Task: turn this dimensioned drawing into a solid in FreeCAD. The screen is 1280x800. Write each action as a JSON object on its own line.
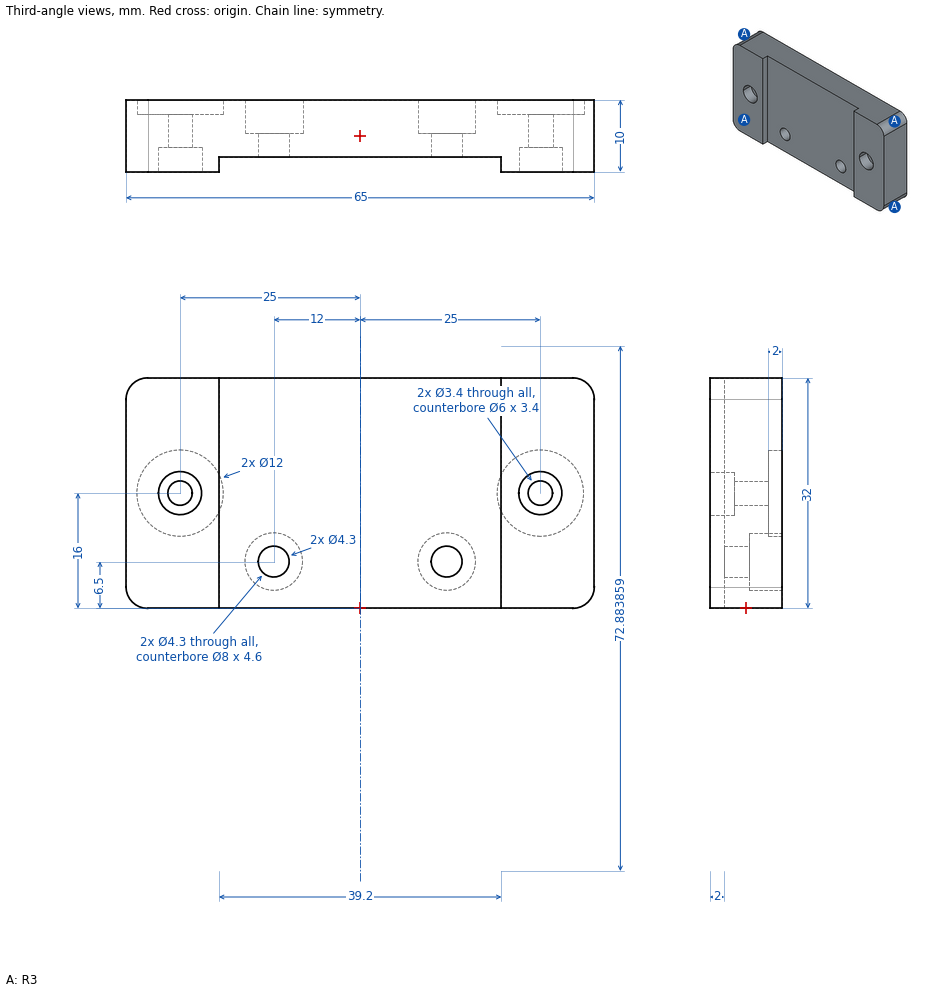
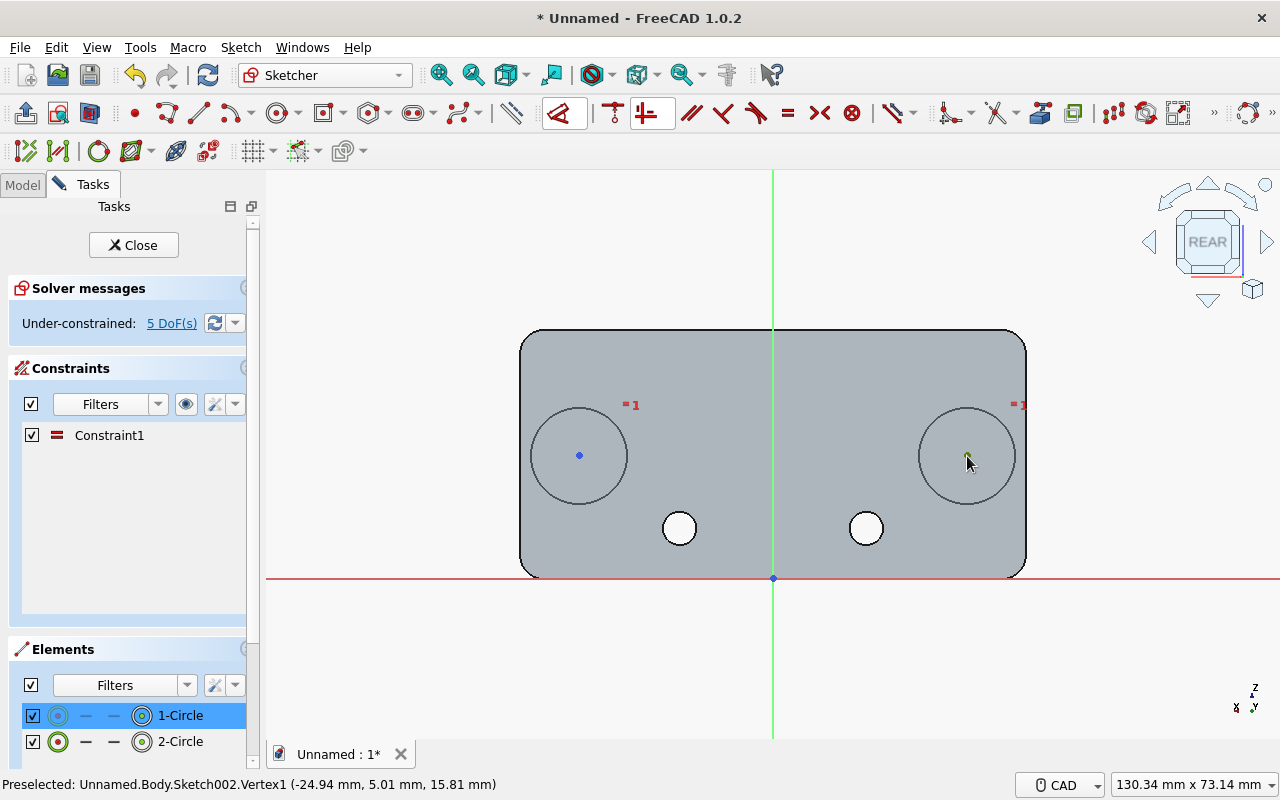
{"action": "left_click", "coordinate": [579, 456]}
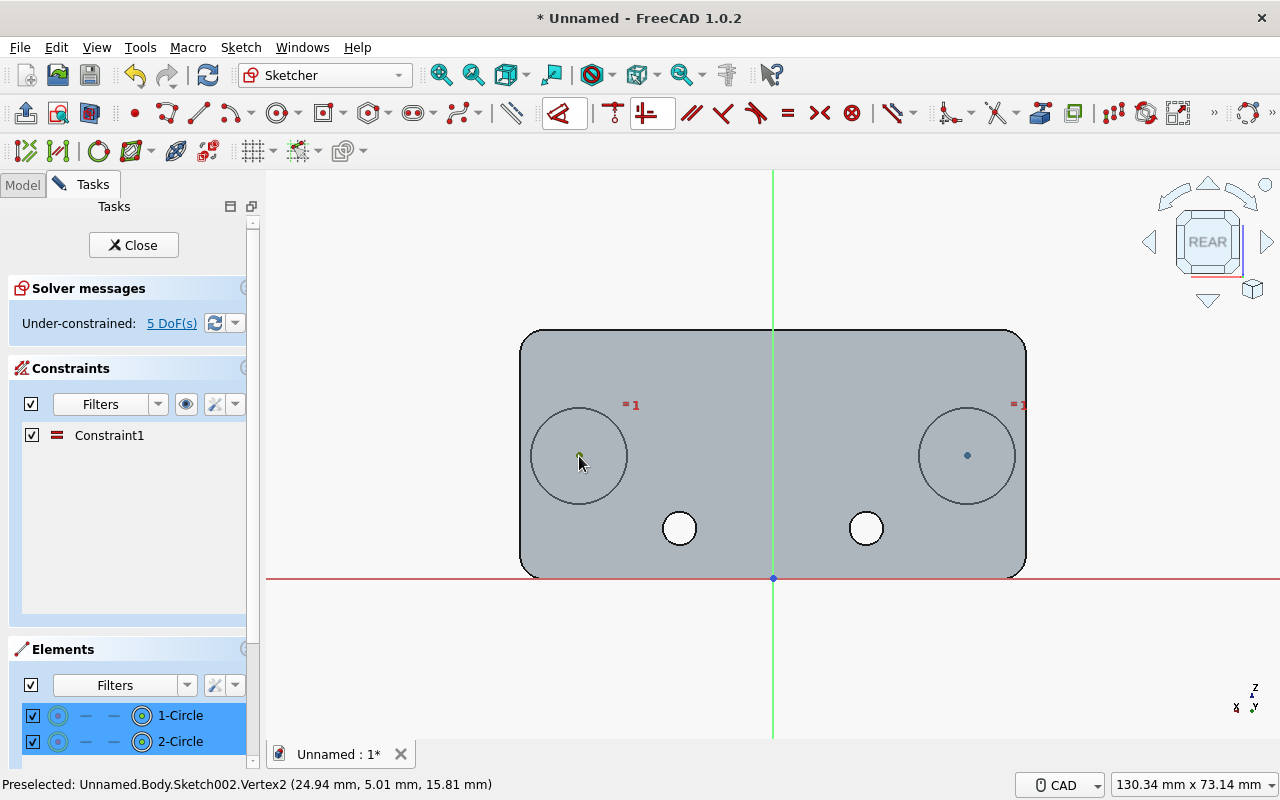
{"action": "left_click", "coordinate": [773, 674]}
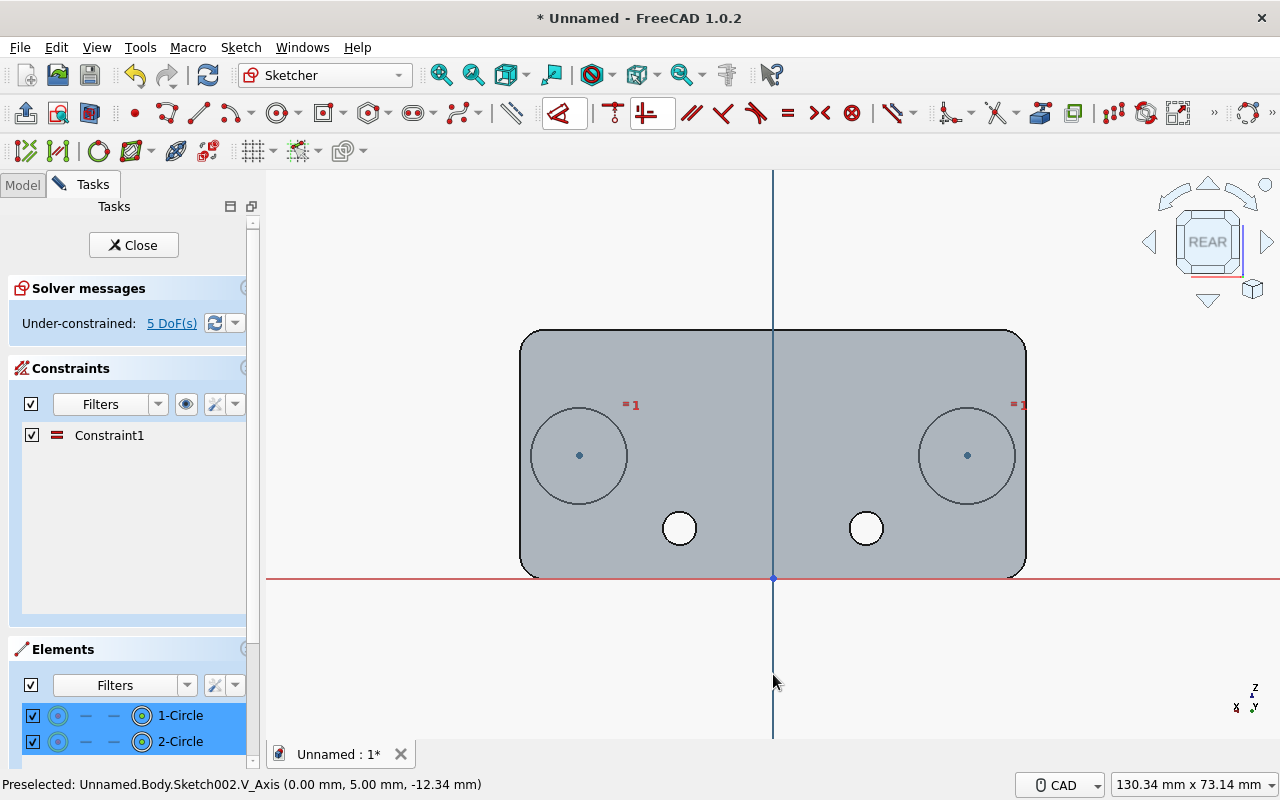
{"action": "left_click", "coordinate": [820, 114]}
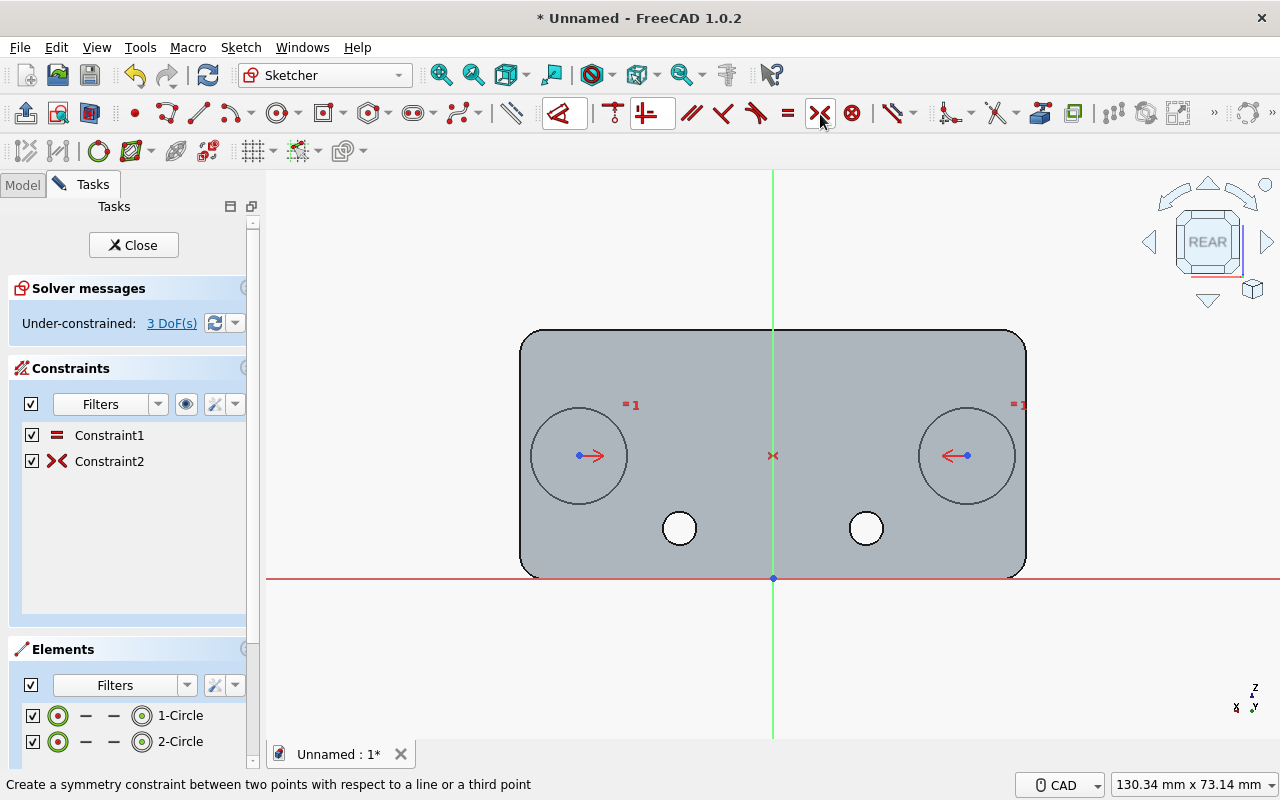
{"action": "left_click", "coordinate": [1001, 422]}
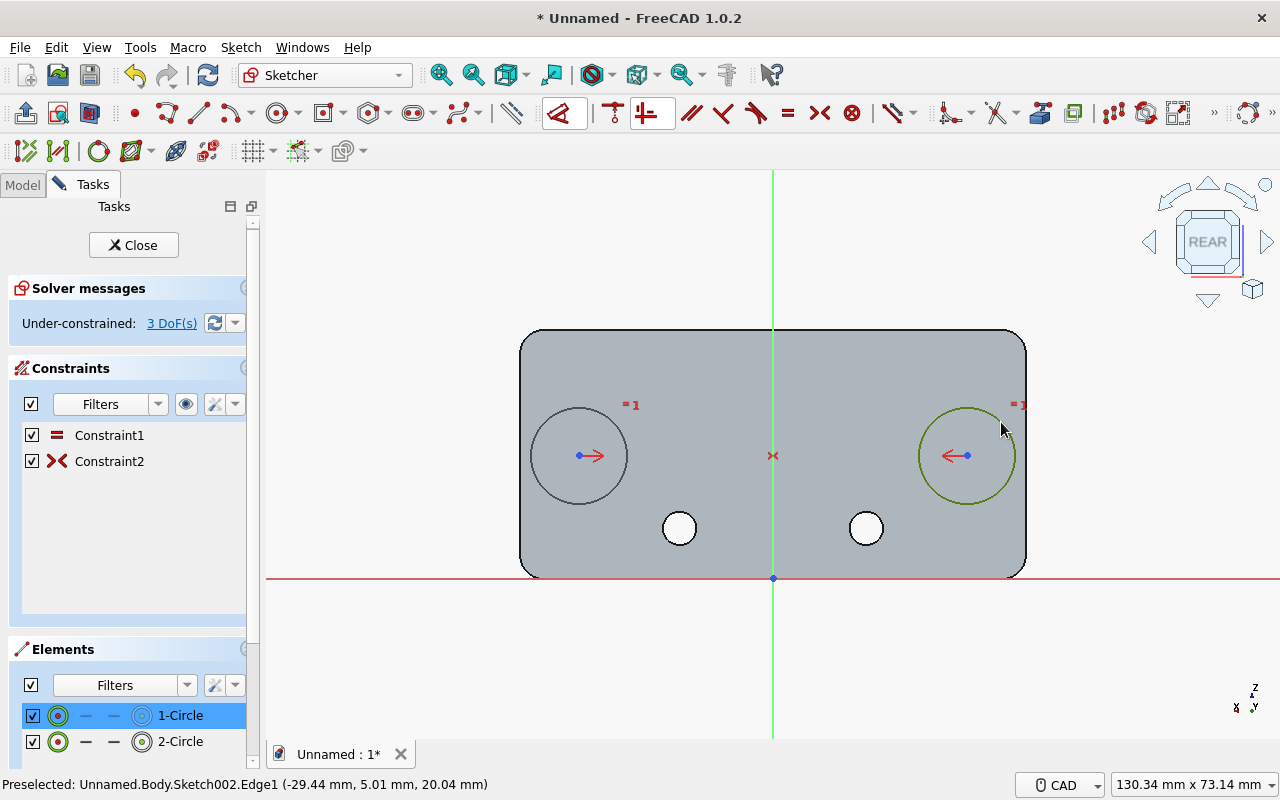
{"action": "left_click", "coordinate": [582, 114]}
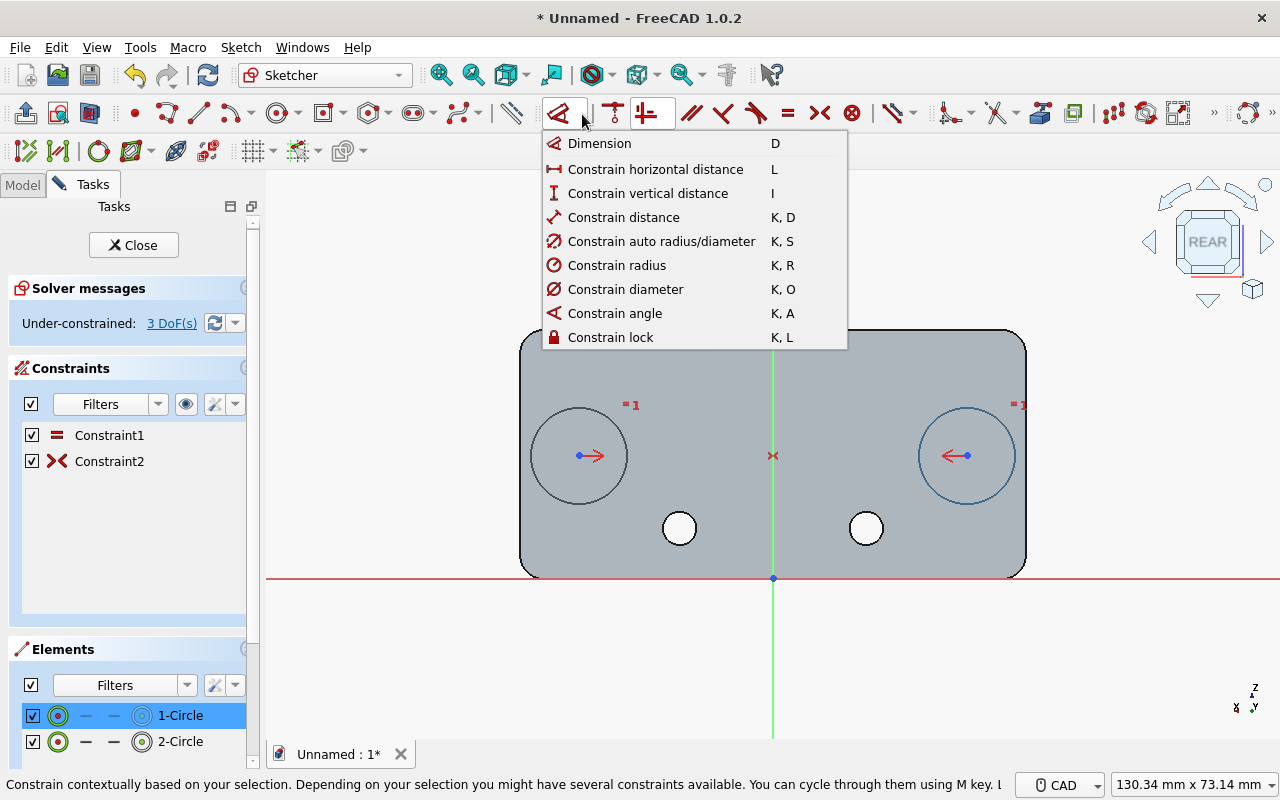
{"action": "left_click", "coordinate": [695, 289]}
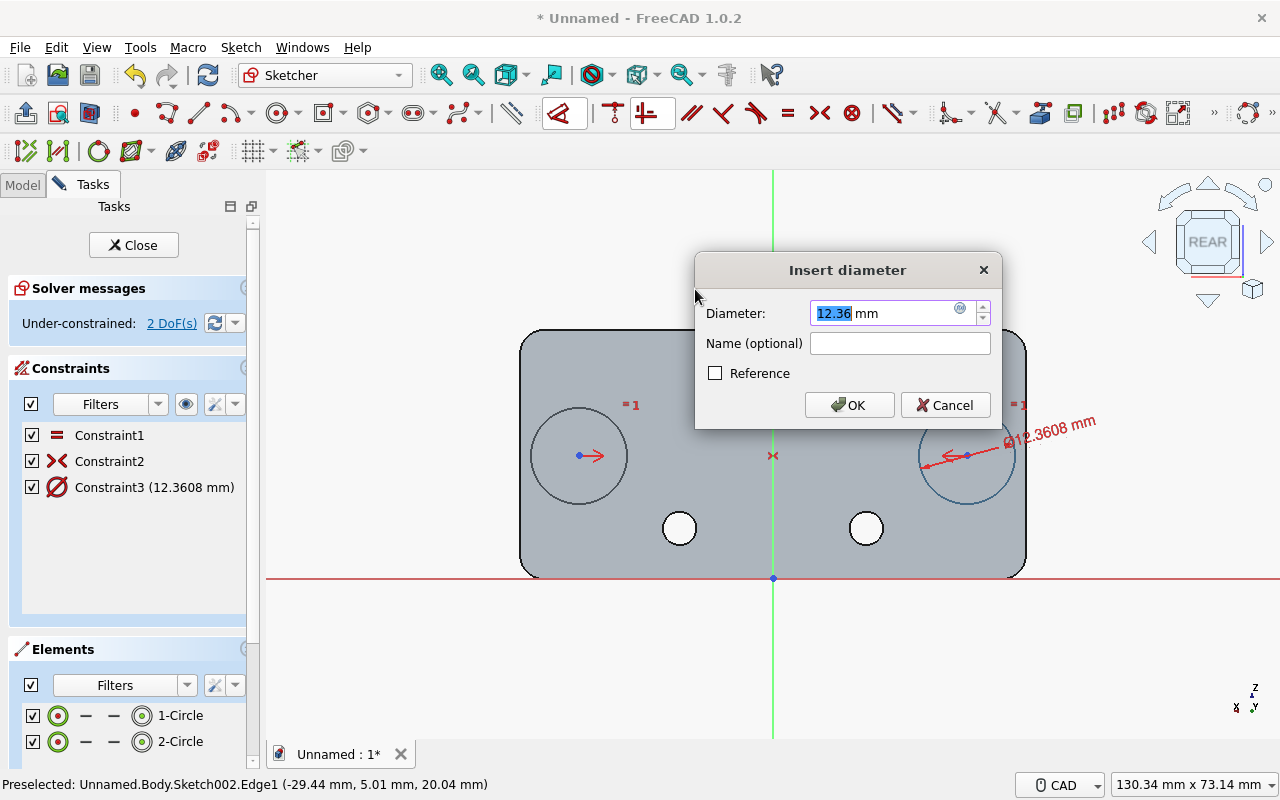
{"action": "type", "text": "12"}
{"action": "key", "text": "Return"}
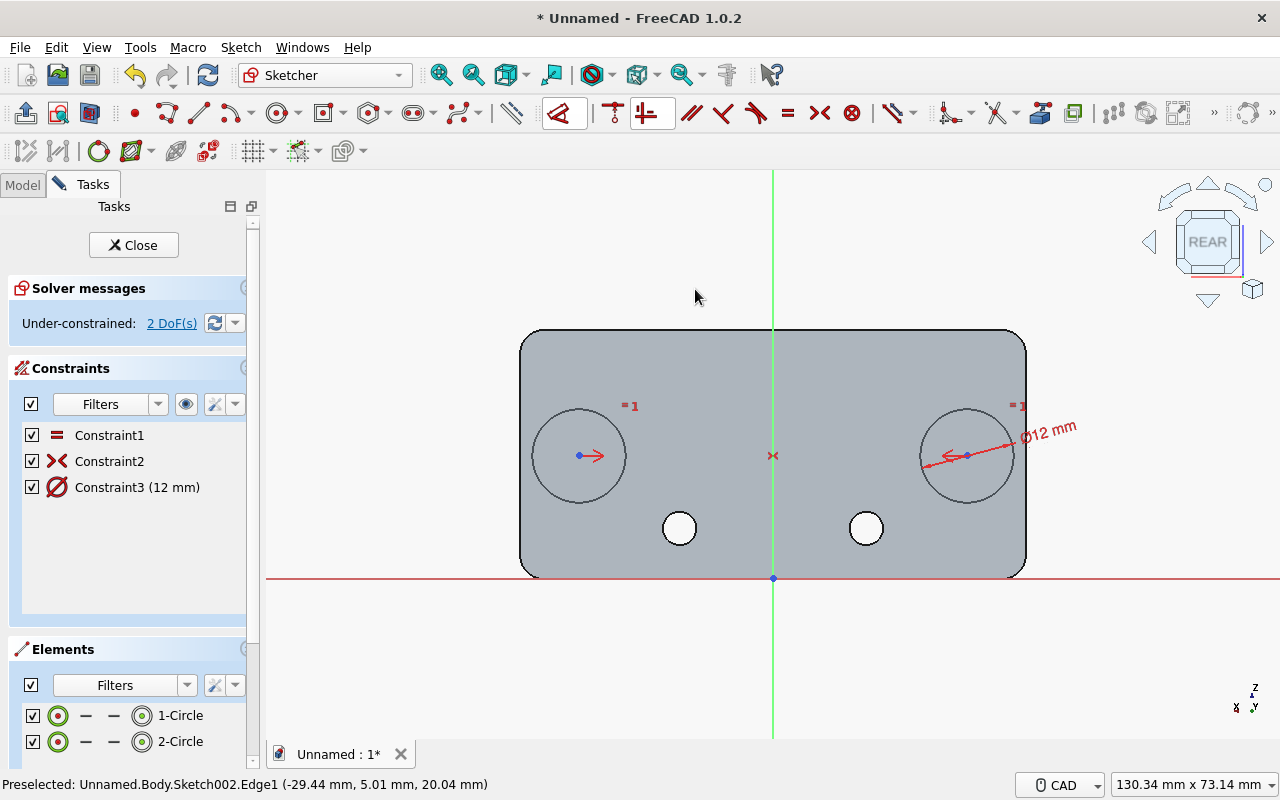
{"action": "left_click", "coordinate": [967, 456]}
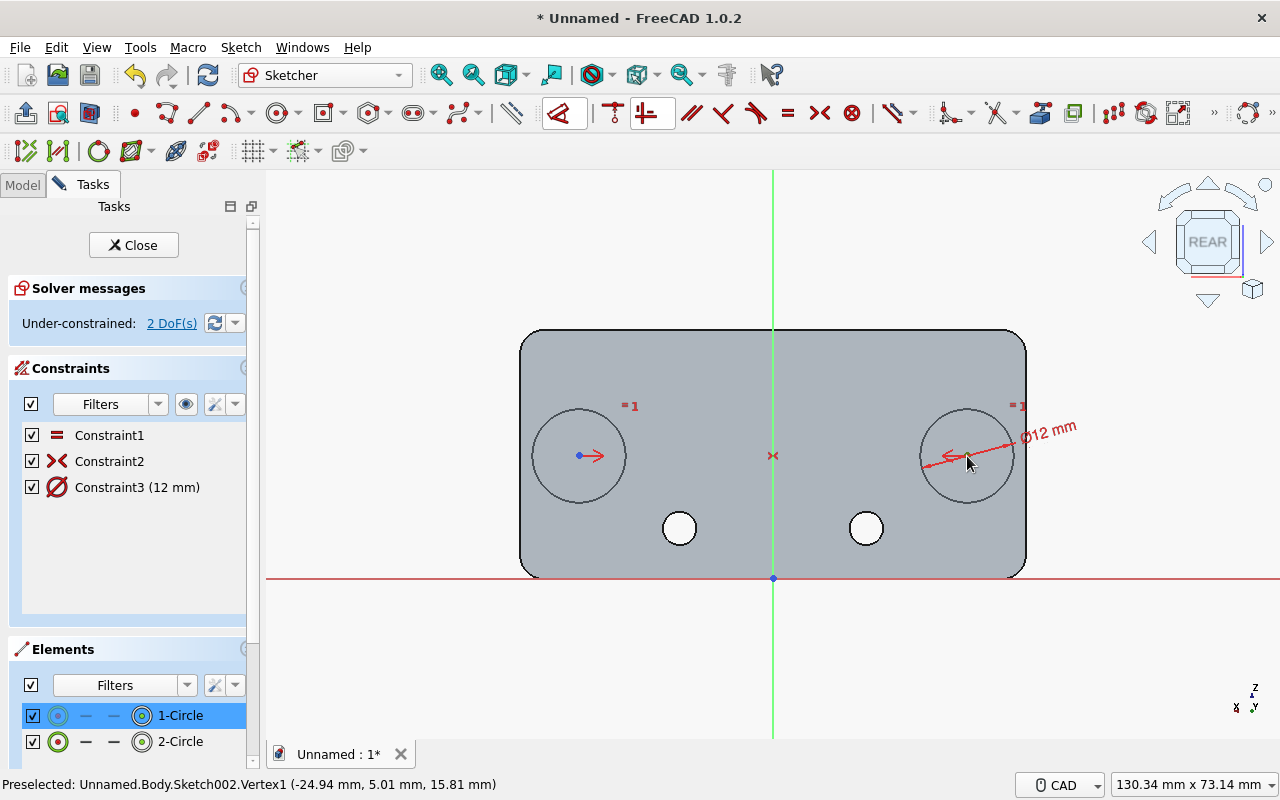
{"action": "key", "text": "l"}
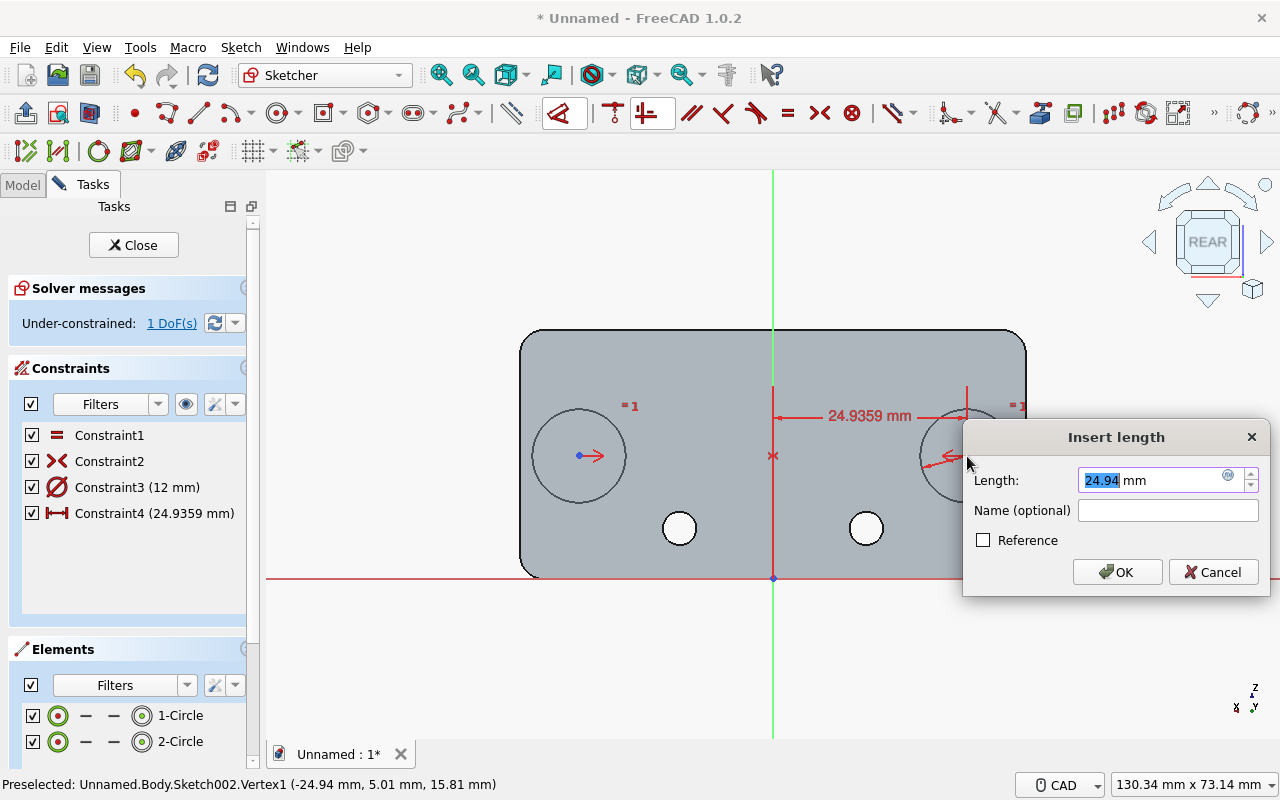
{"action": "type", "text": "25"}
{"action": "key", "text": "Return"}